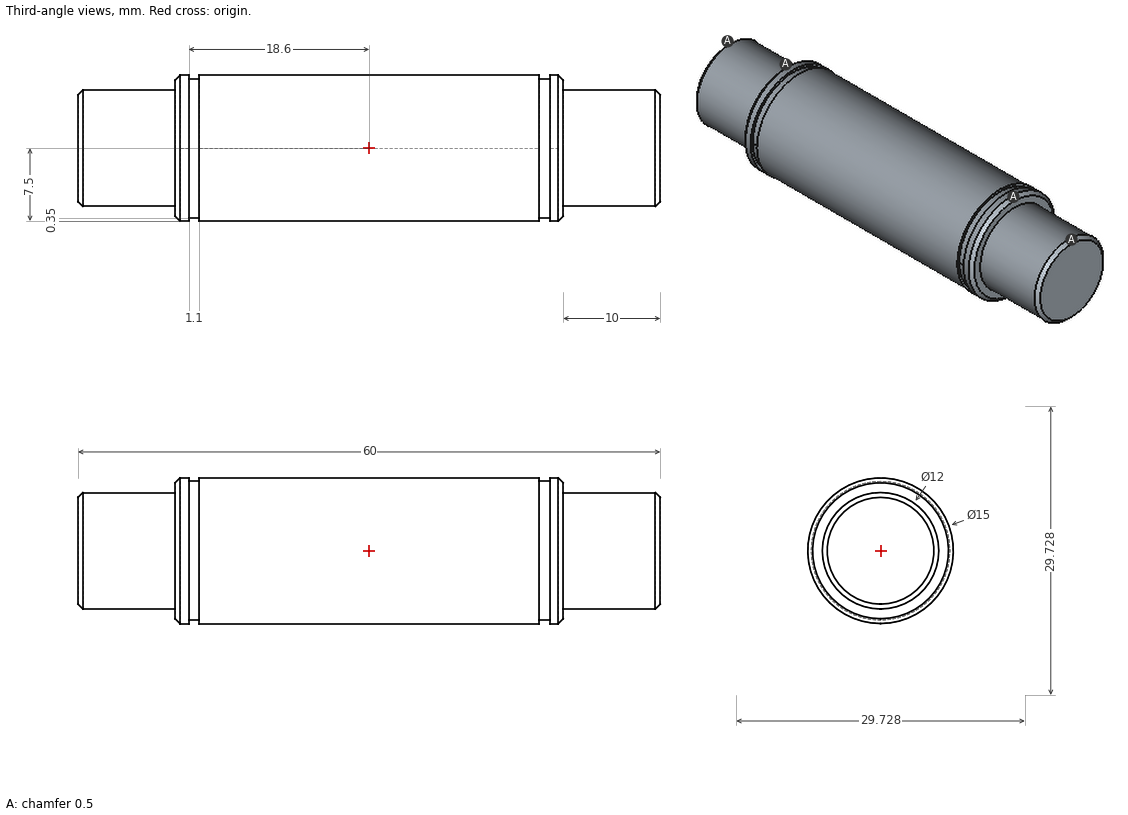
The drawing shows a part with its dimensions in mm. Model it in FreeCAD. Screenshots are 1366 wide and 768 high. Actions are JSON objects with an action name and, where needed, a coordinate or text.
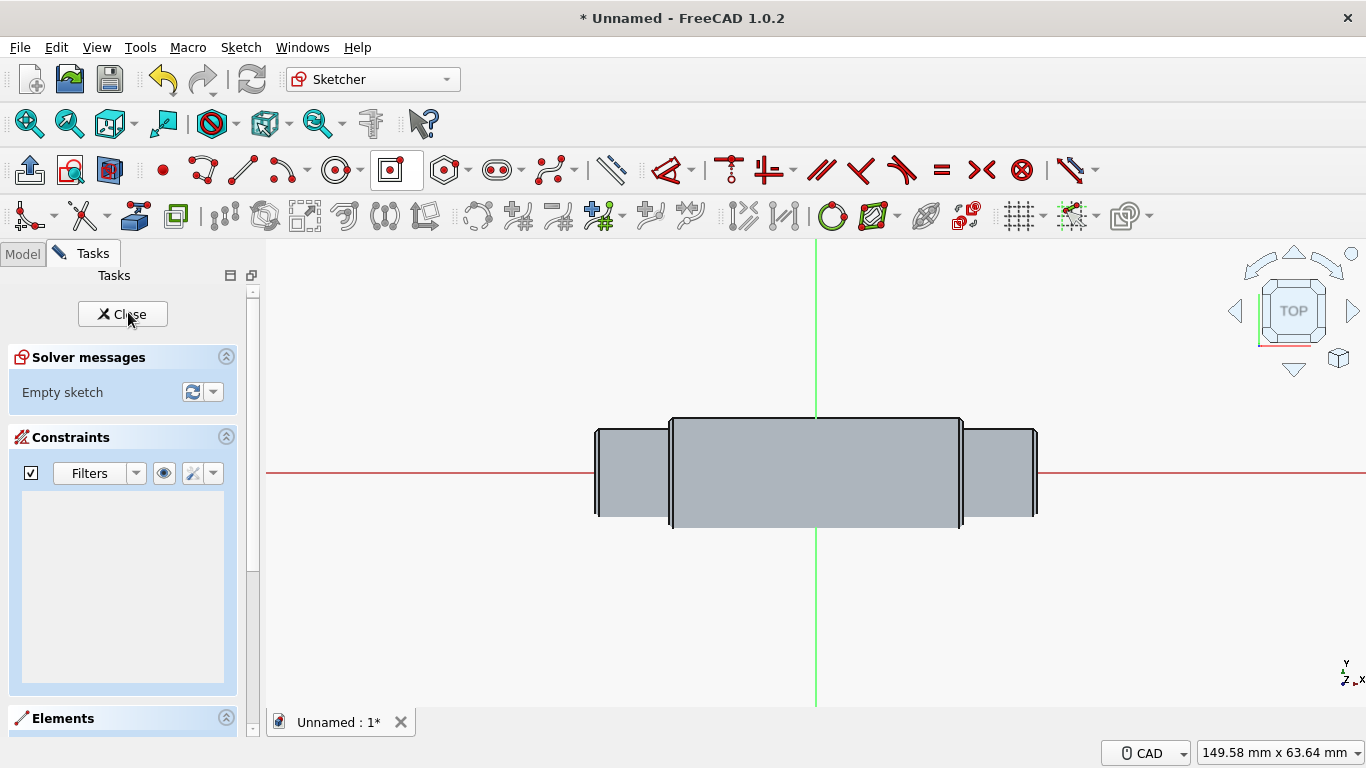
{"action": "key", "text": "q s"}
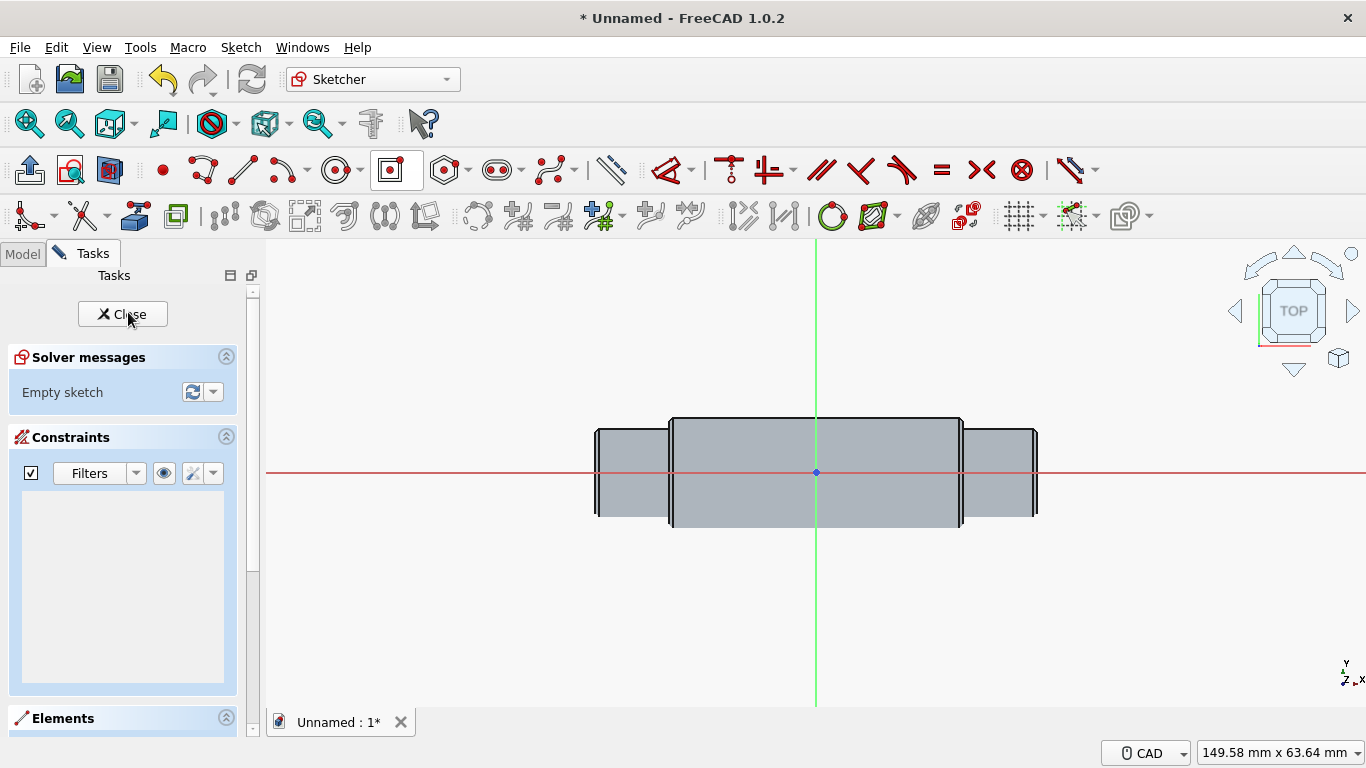
{"action": "scroll", "coordinate": [680, 530], "scroll_direction": "up", "scroll_amount": 15}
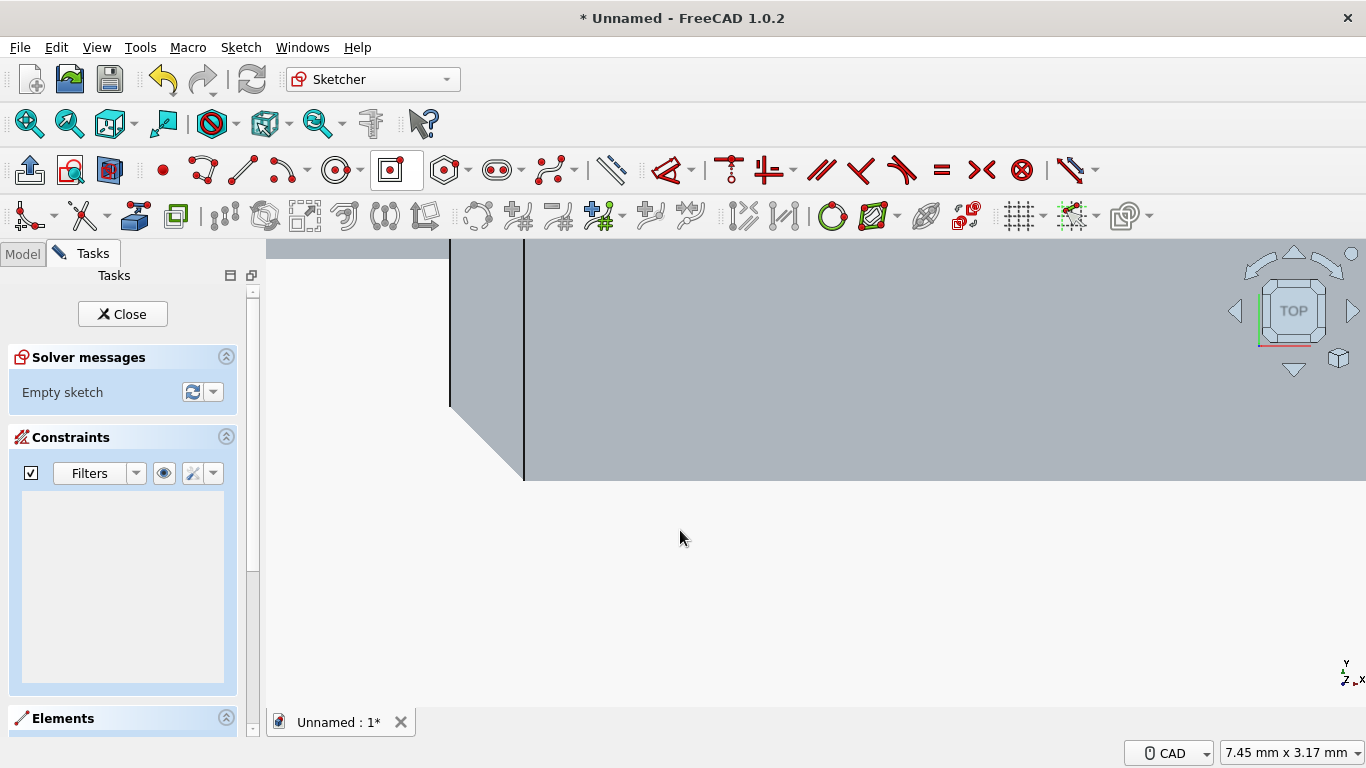
{"action": "scroll", "coordinate": [735, 449], "scroll_direction": "up", "scroll_amount": 7}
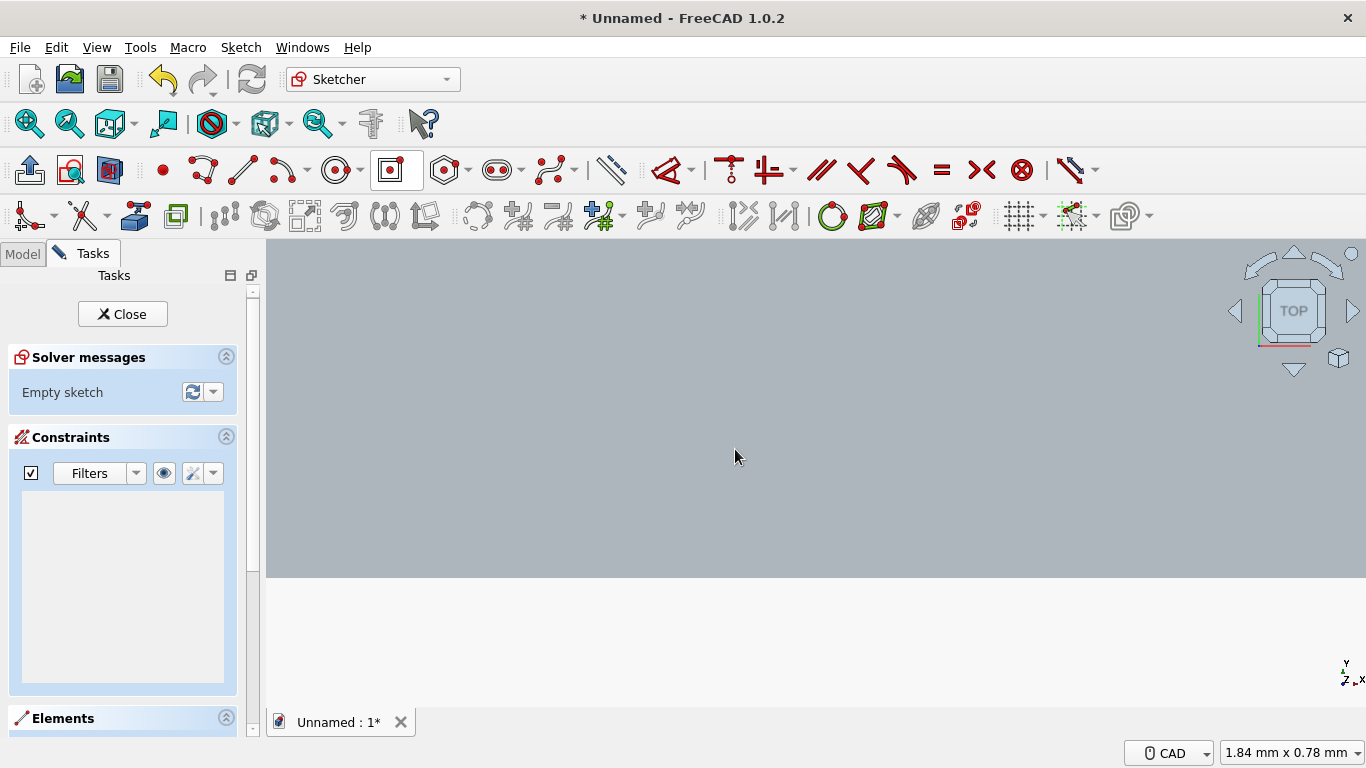
{"action": "key", "text": "g r"}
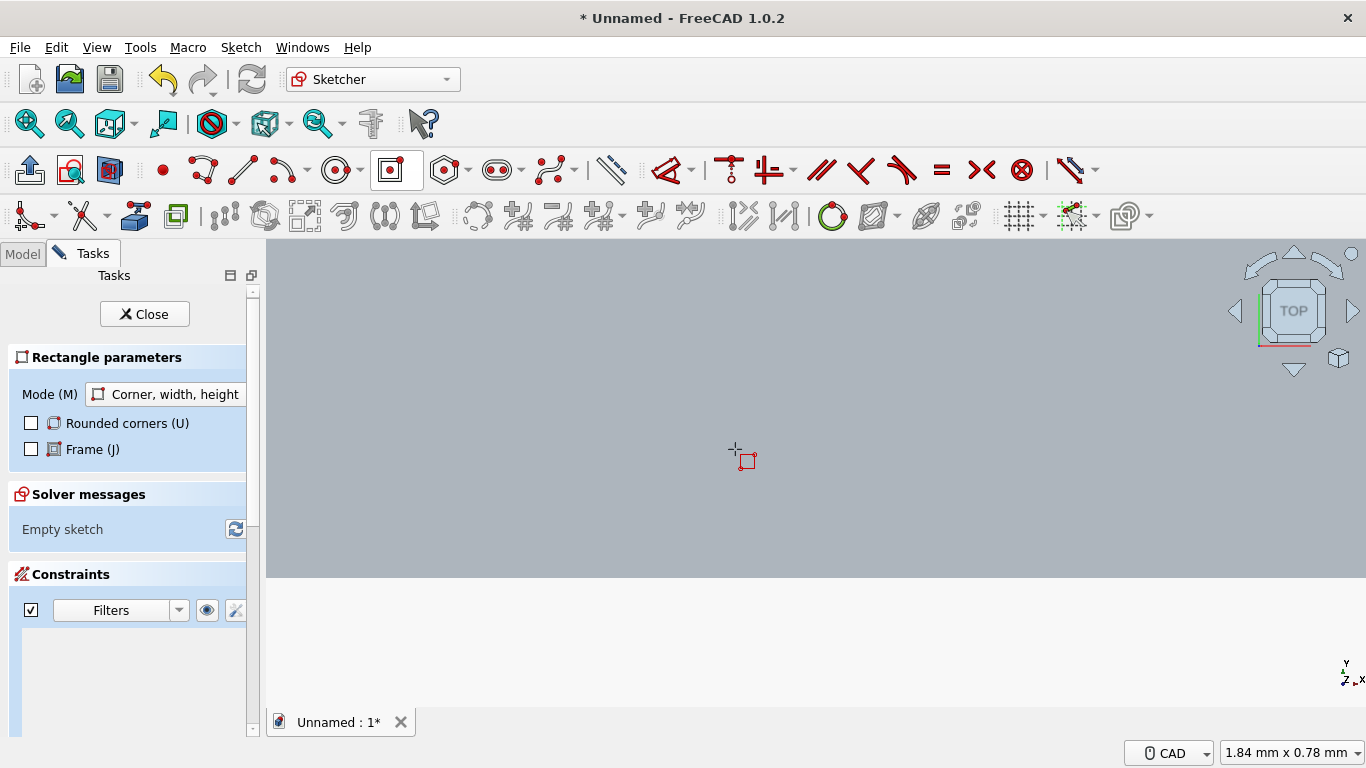
{"action": "left_click", "coordinate": [418, 368]}
{"action": "left_click", "coordinate": [1077, 578]}
{"action": "key", "text": "Escape"}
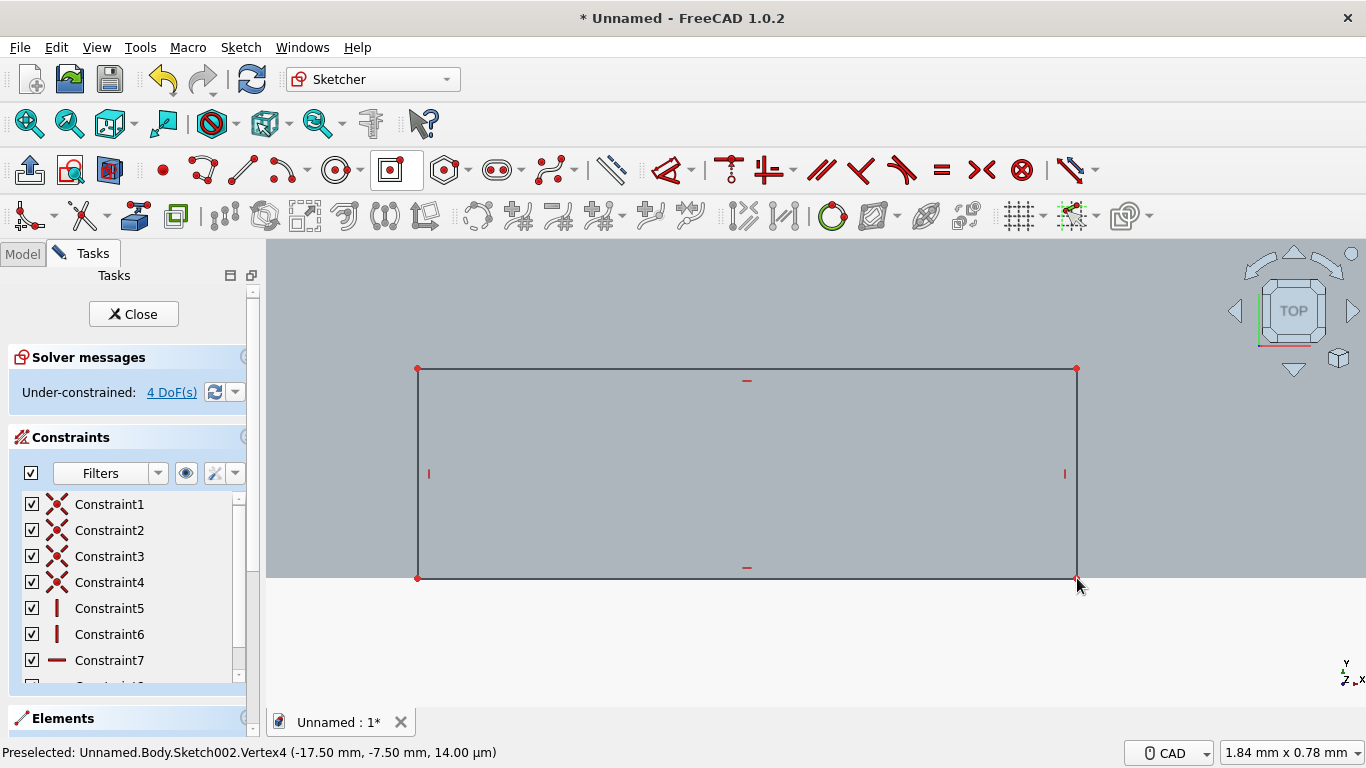
{"action": "key", "text": "d"}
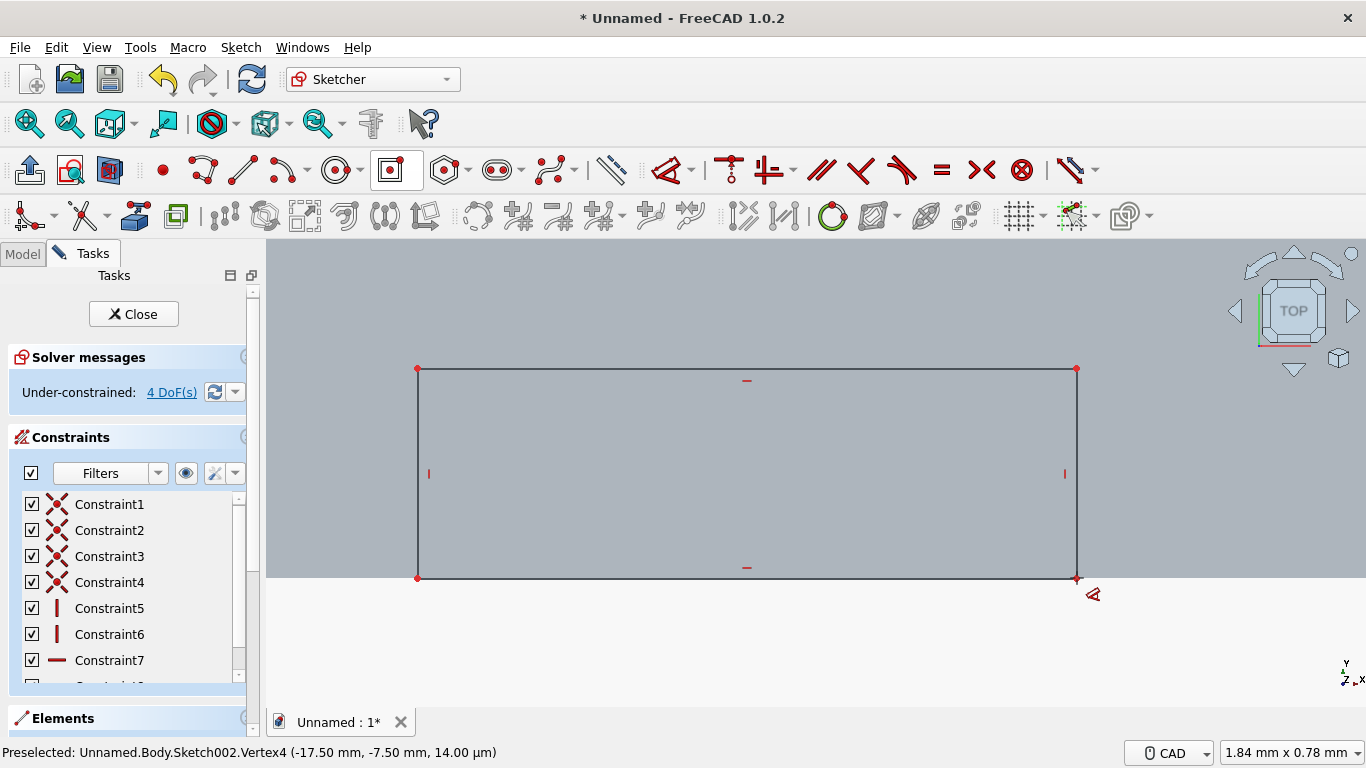
{"action": "left_click", "coordinate": [616, 579]}
{"action": "left_click", "coordinate": [747, 613]}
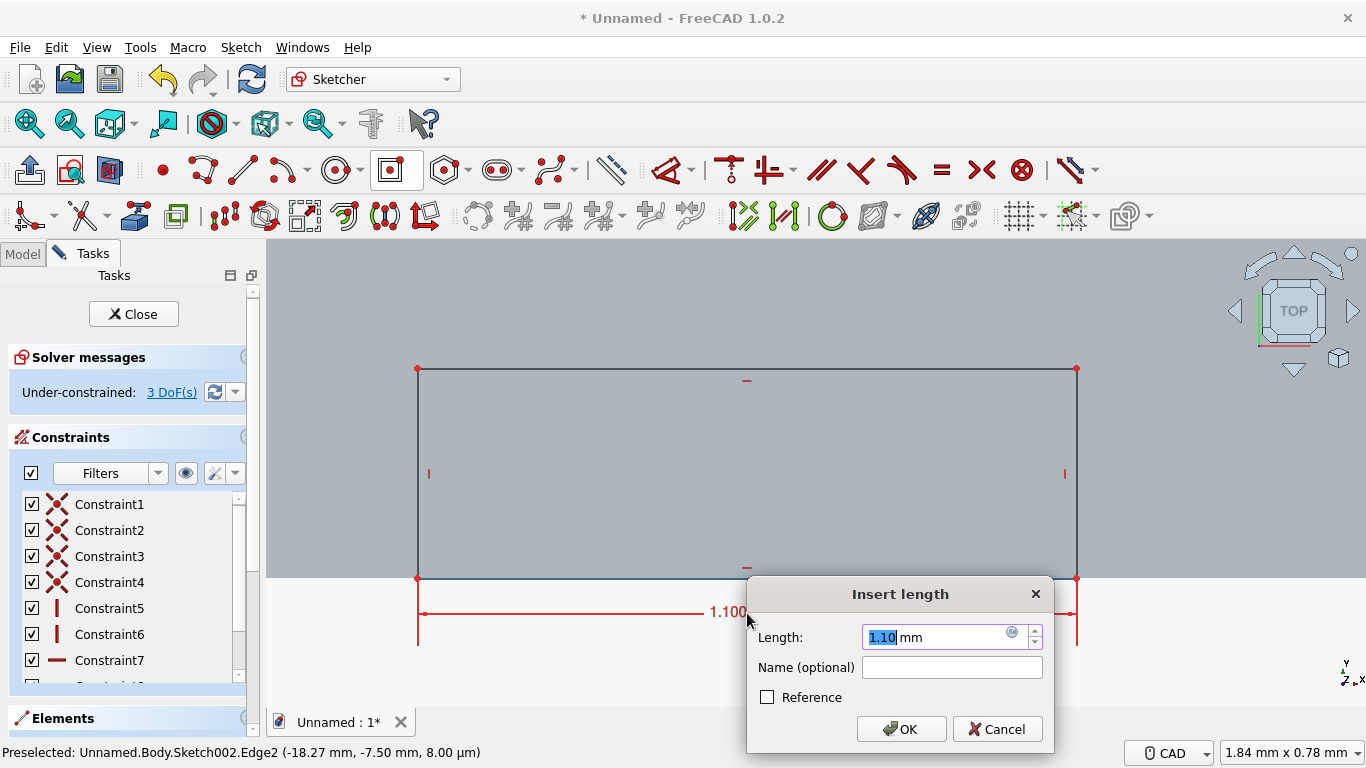
{"action": "type", "text": "1.1"}
{"action": "key", "text": "Return"}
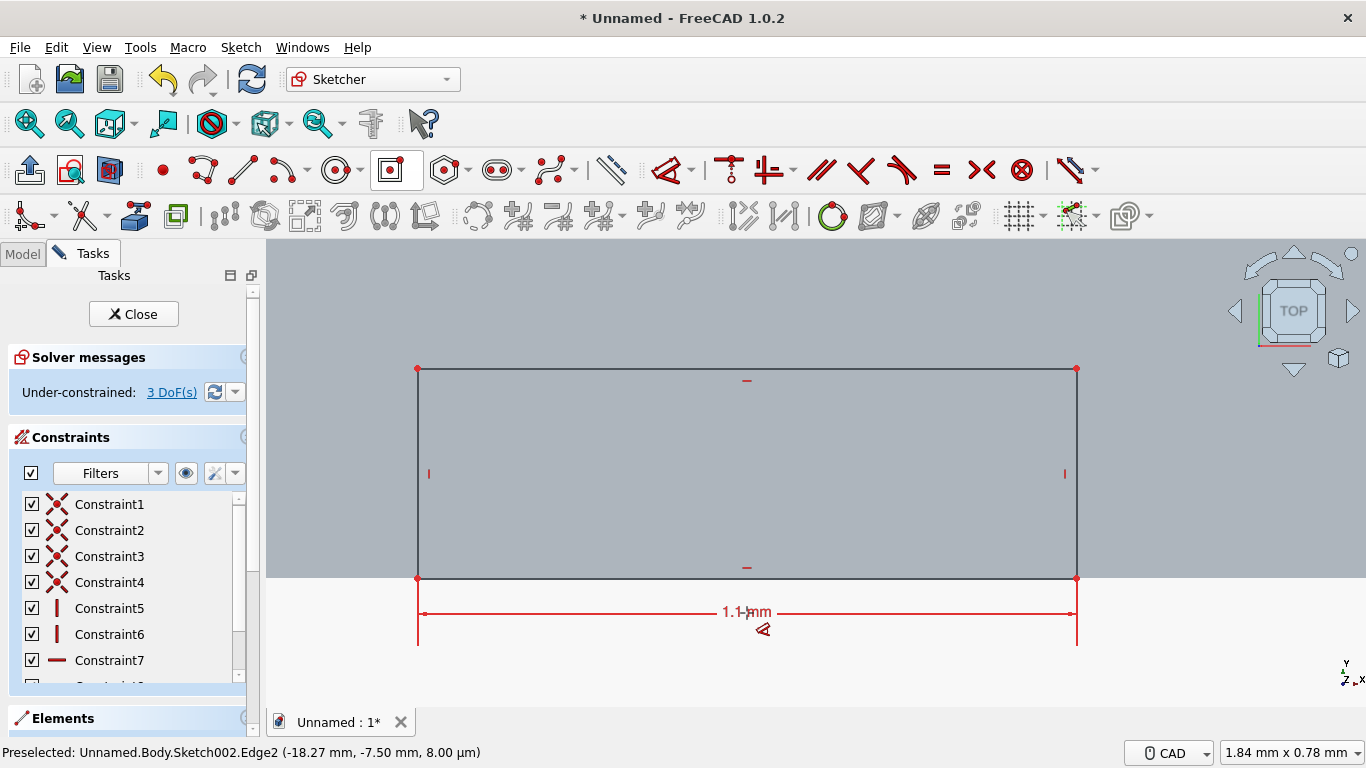
{"action": "left_click", "coordinate": [418, 432]}
{"action": "left_click", "coordinate": [384, 474]}